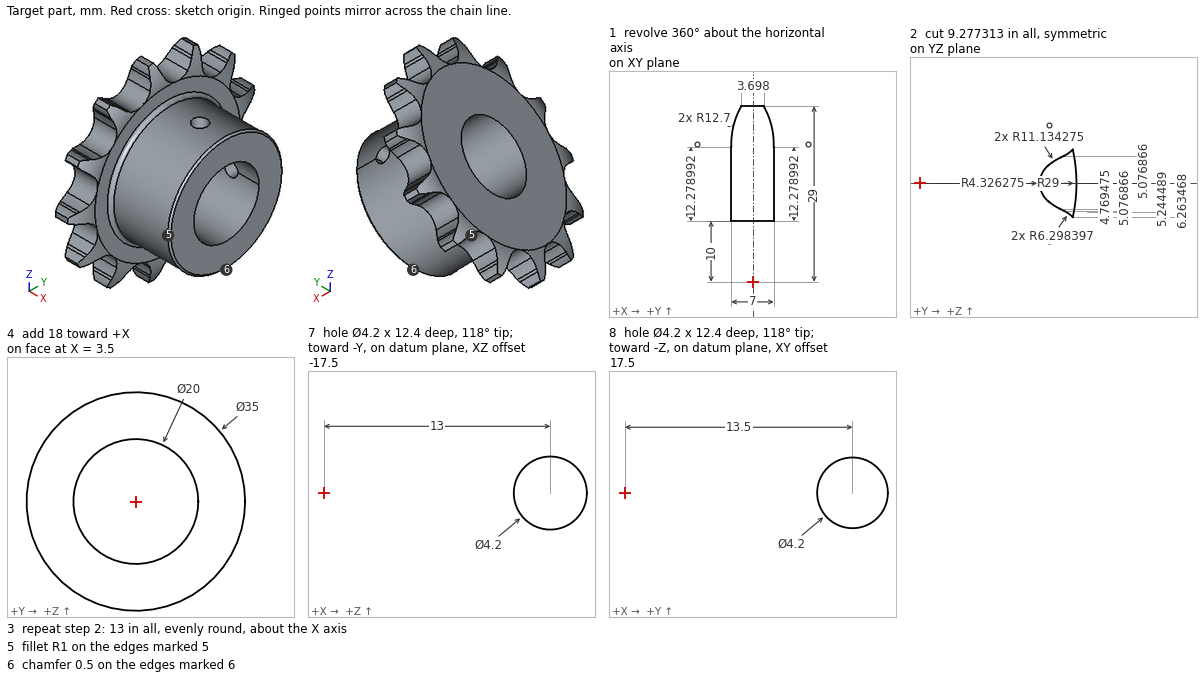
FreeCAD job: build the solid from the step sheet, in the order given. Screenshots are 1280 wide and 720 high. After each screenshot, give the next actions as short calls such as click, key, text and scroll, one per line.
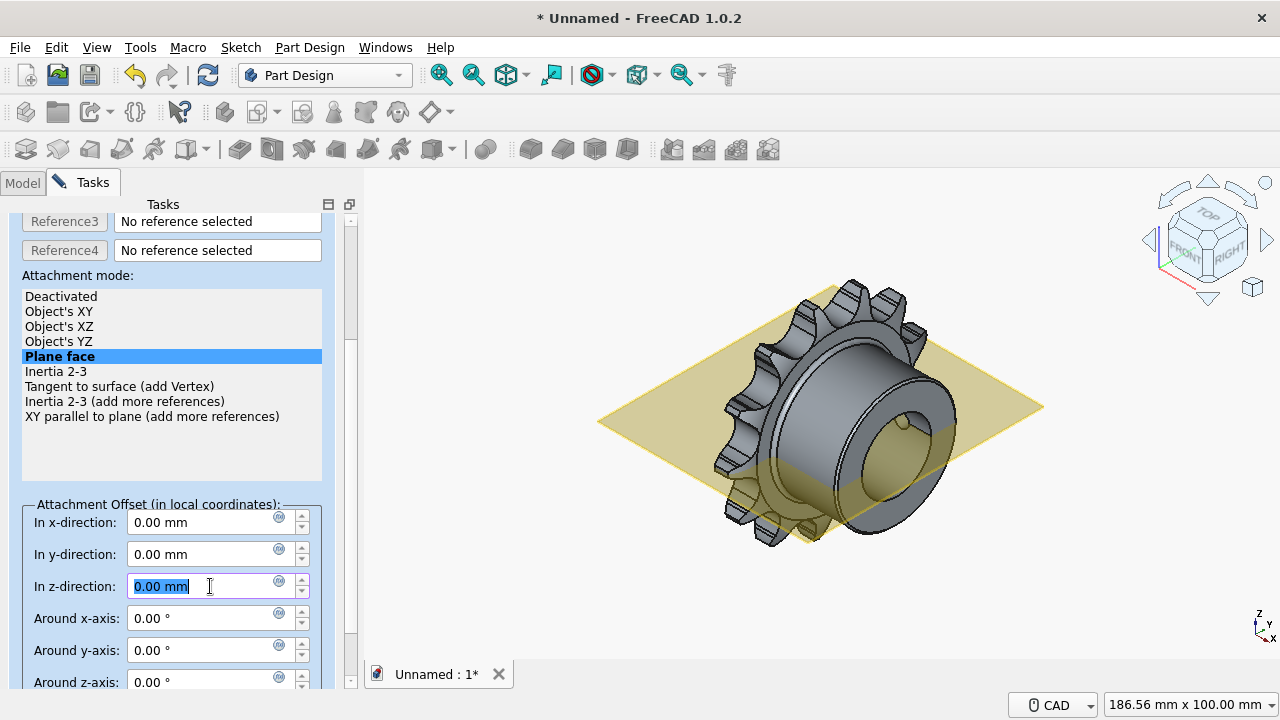
text(17.5)
key(Tab)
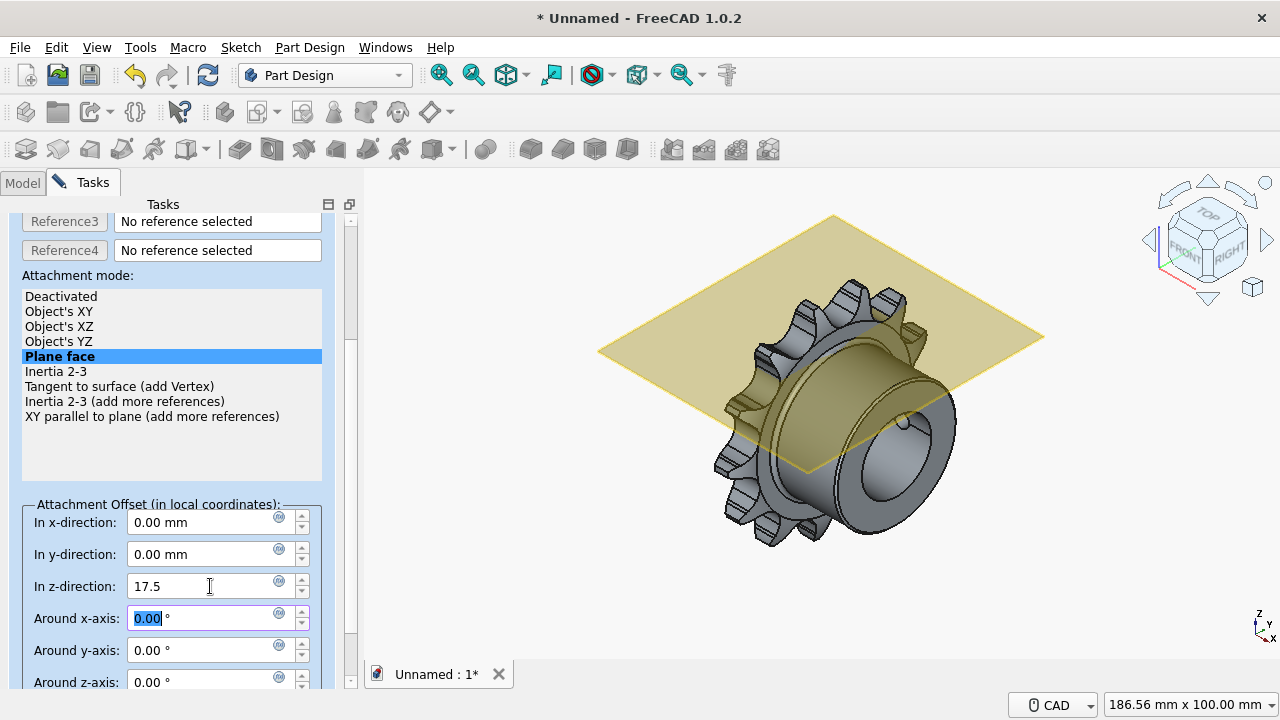
scroll(351, 451, up, 4)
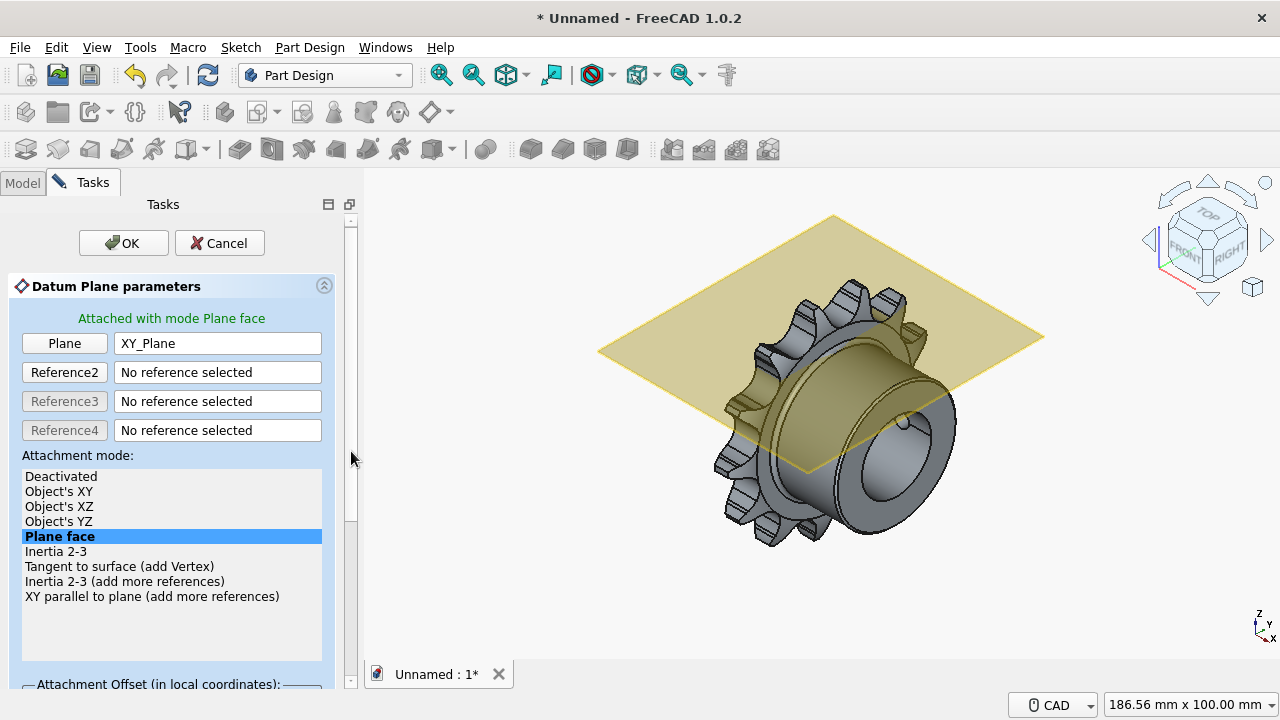
click(124, 243)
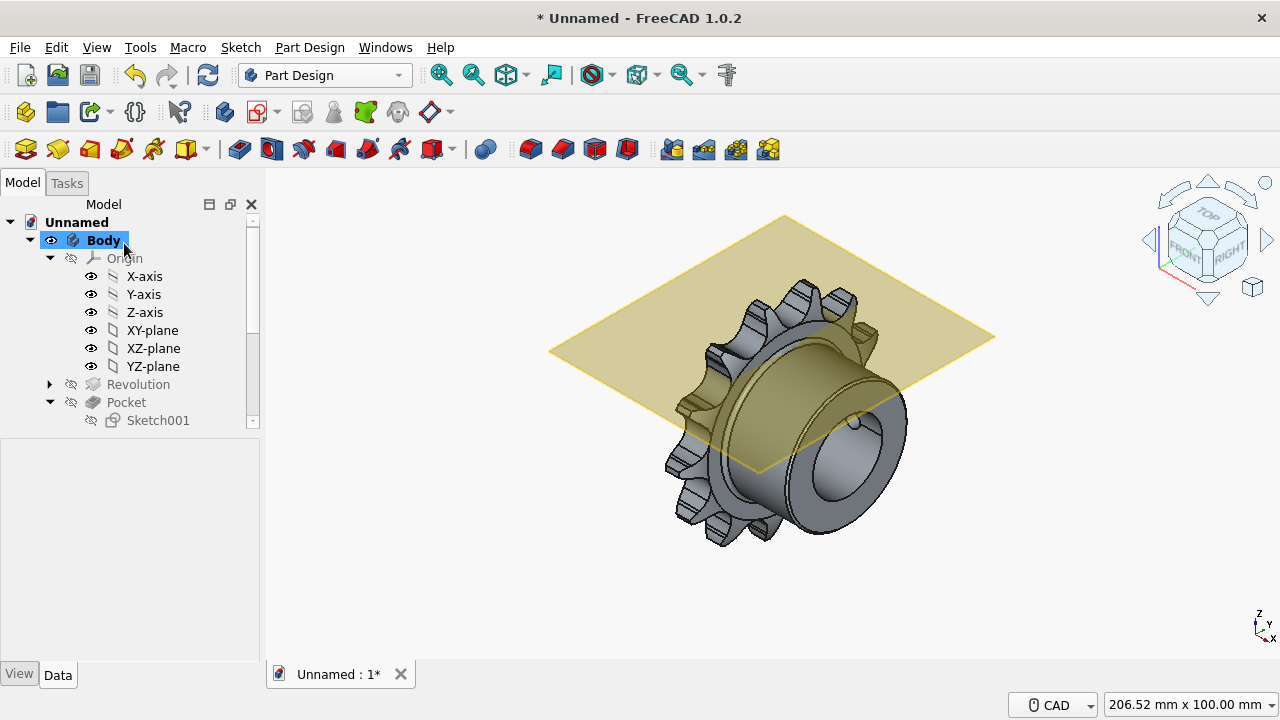
scroll(100, 326, down, 3)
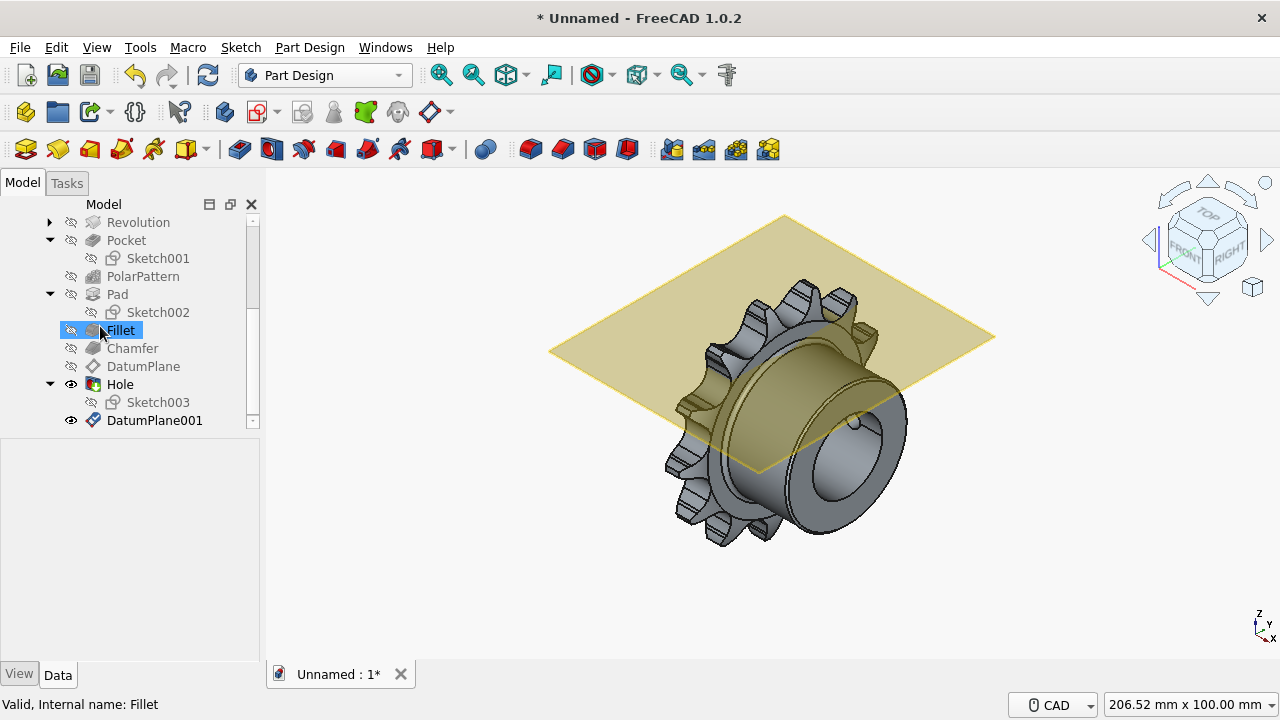
click(116, 420)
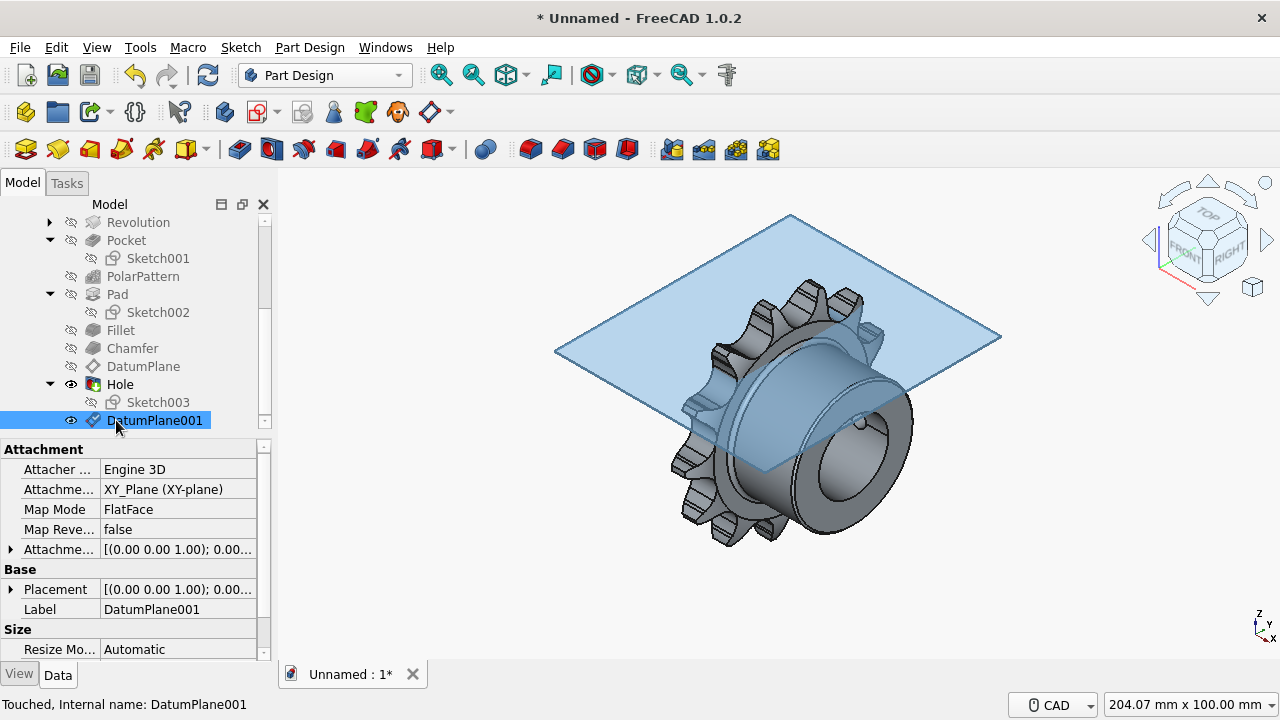
click(258, 112)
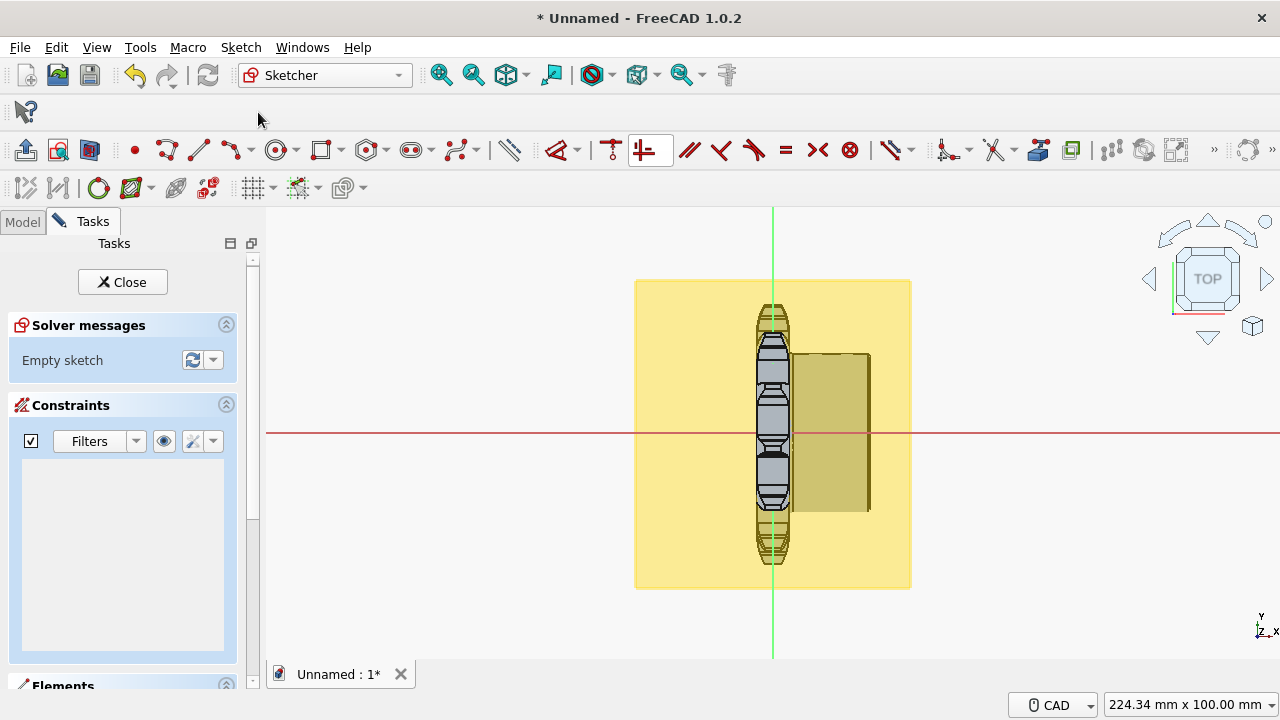
click(90, 150)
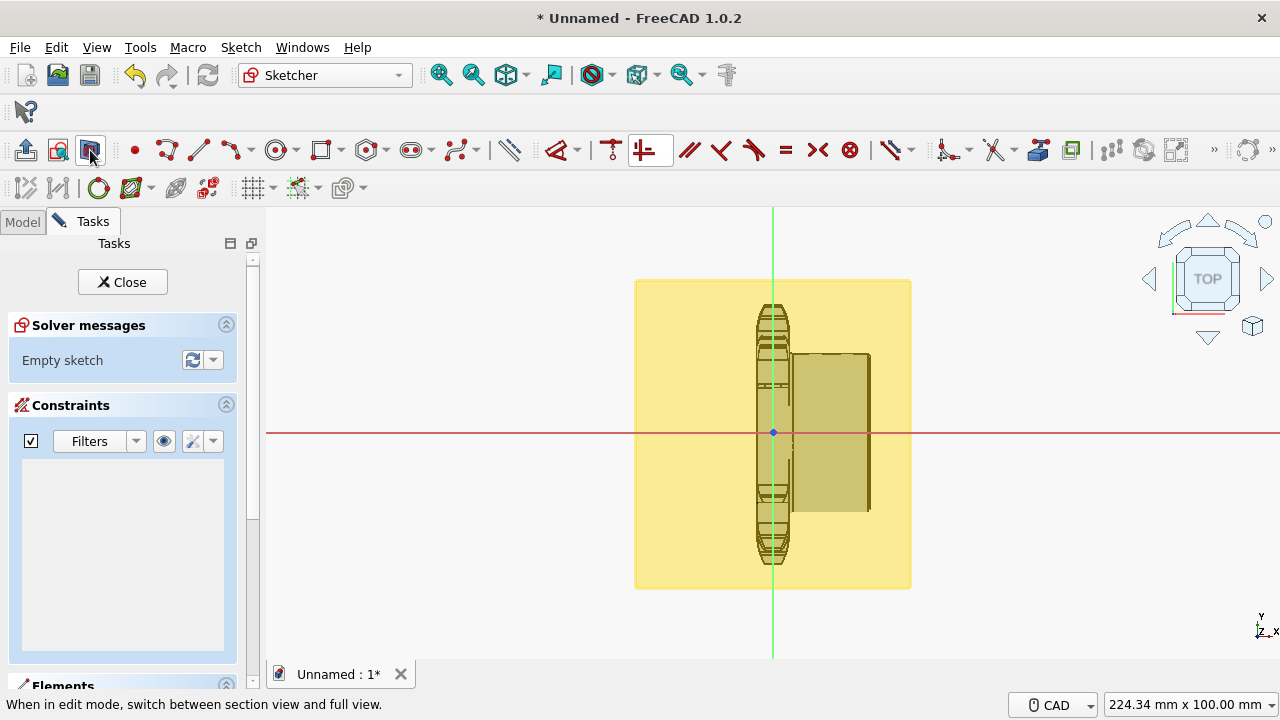
scroll(844, 433, up, 13)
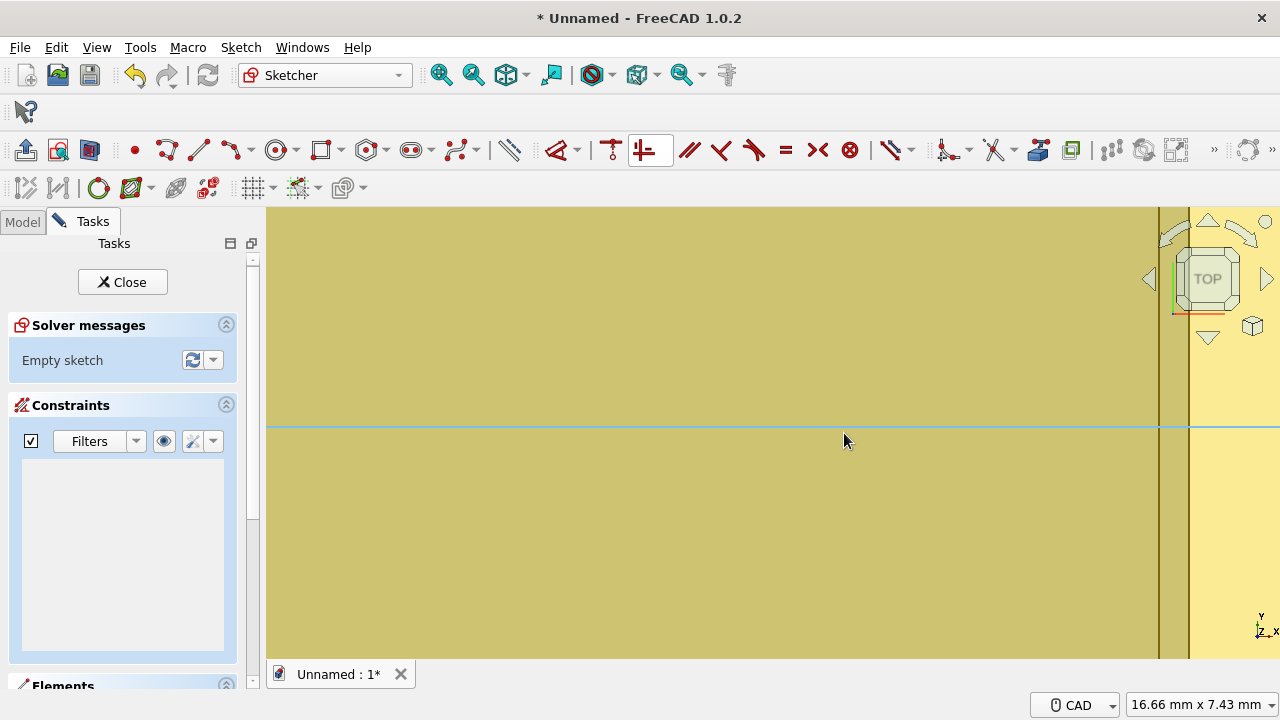
click(276, 150)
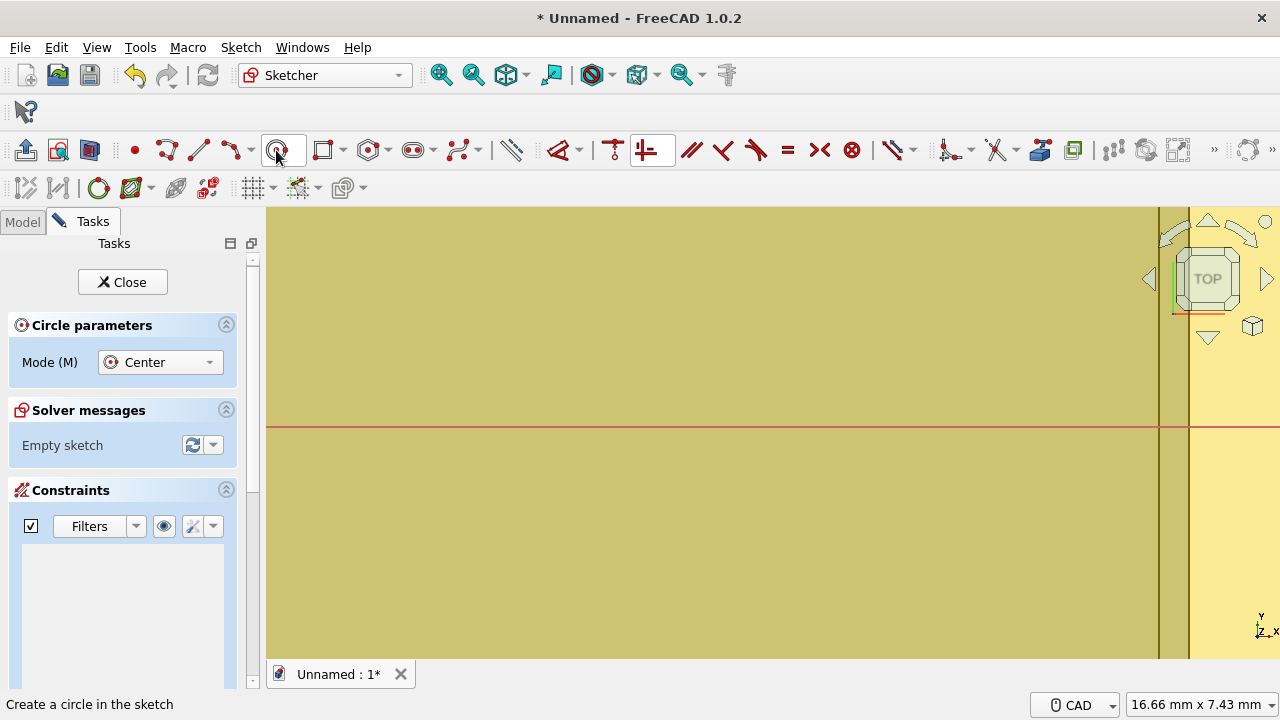
click(703, 427)
move(793, 336)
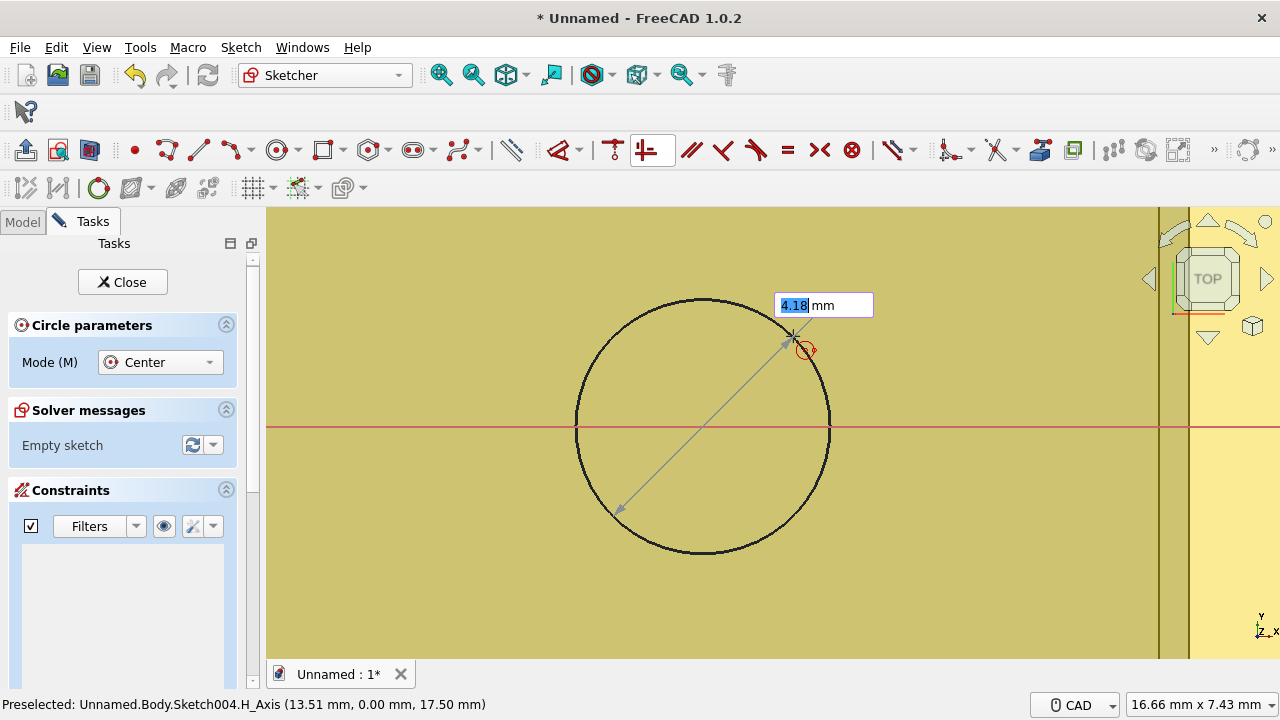
text(4.2)
key(Return)
key(Escape)